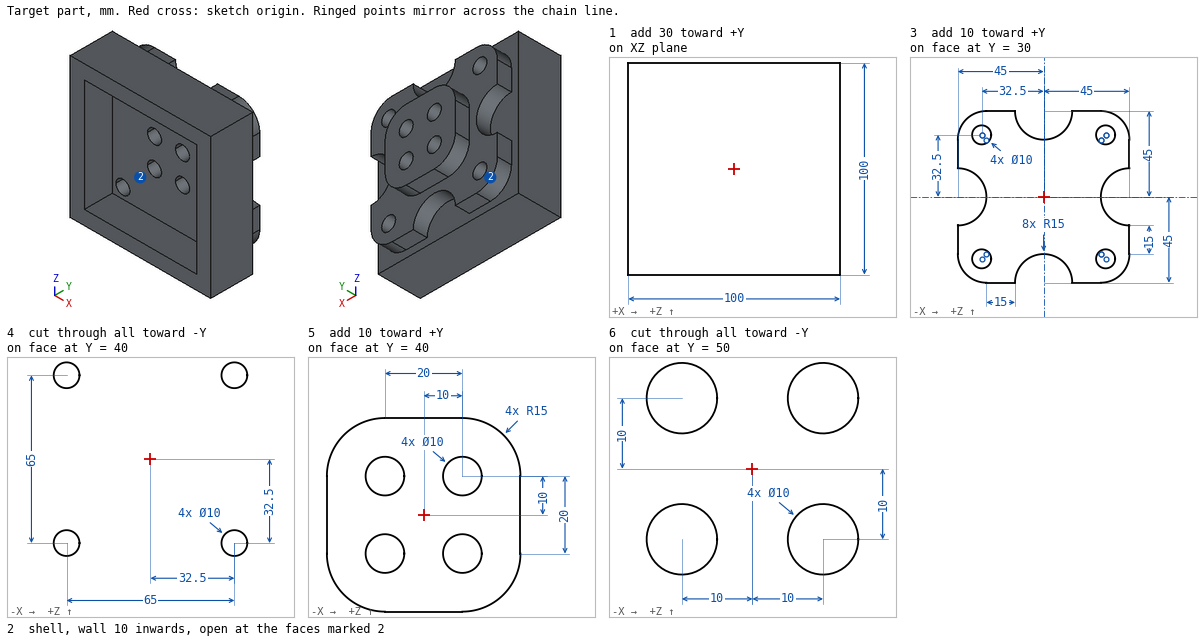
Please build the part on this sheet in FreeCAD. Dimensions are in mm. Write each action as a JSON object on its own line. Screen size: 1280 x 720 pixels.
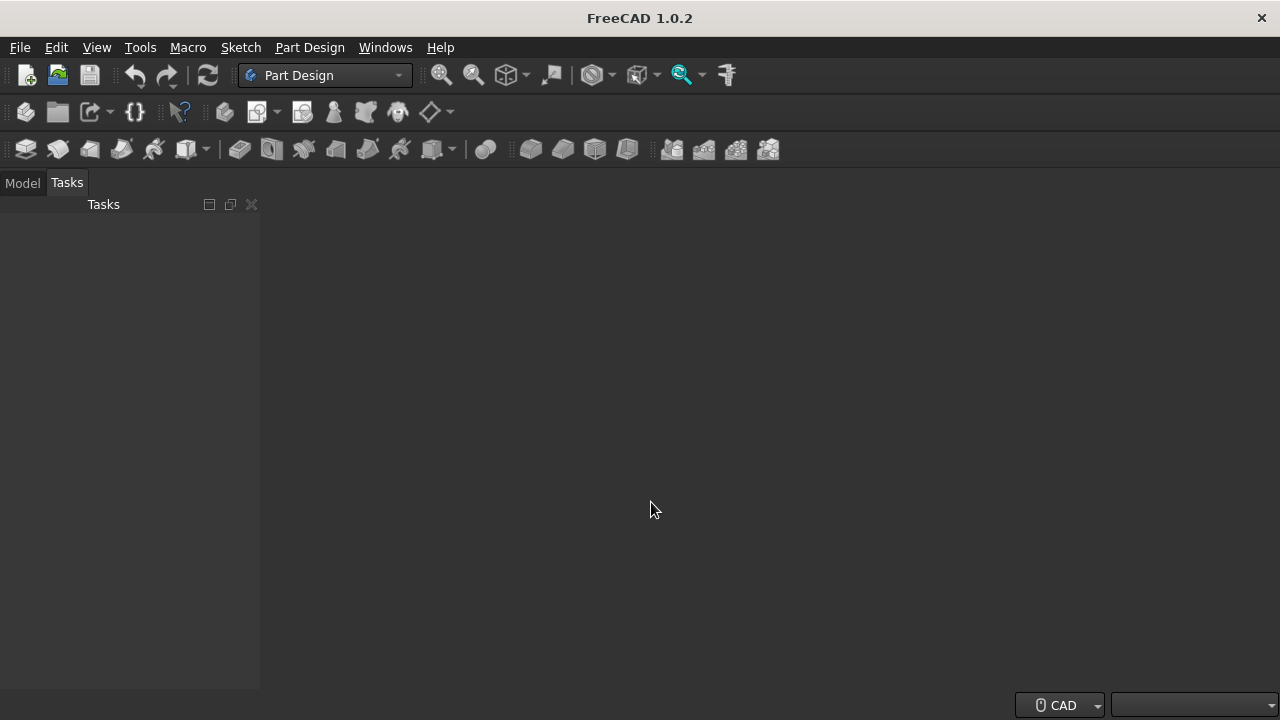
{"action": "left_click", "coordinate": [26, 76]}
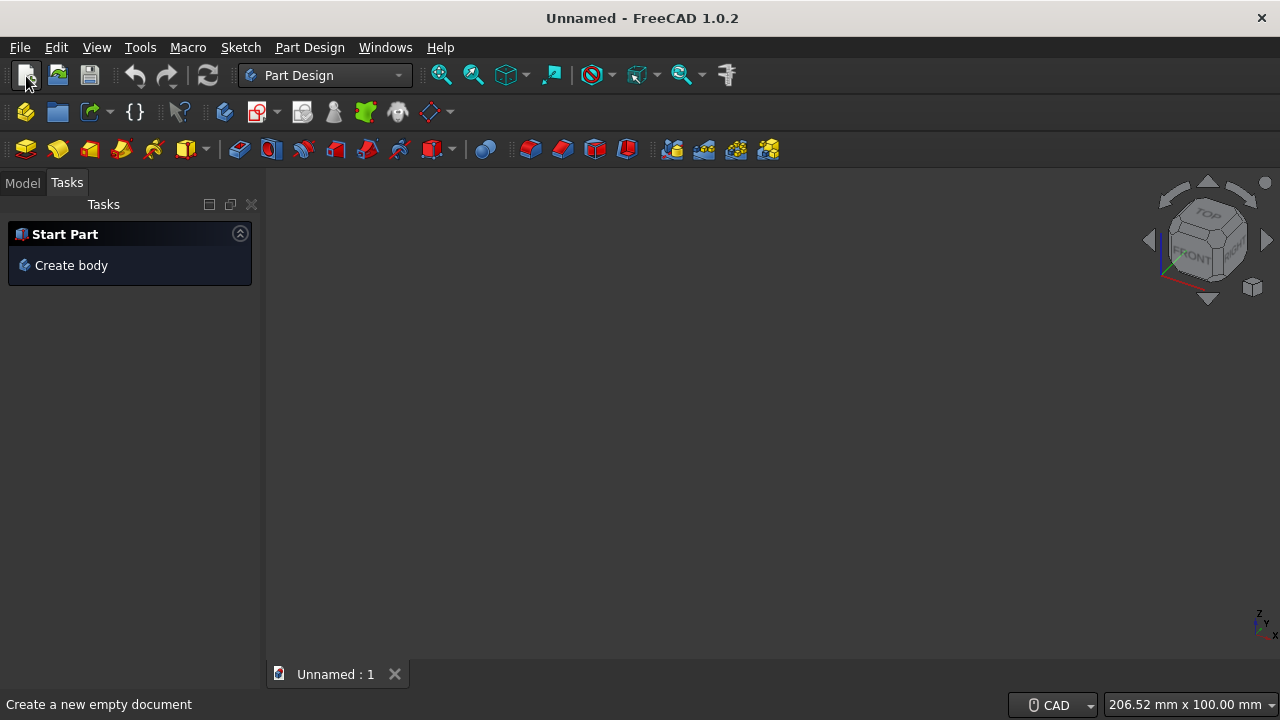
{"action": "left_click", "coordinate": [258, 112]}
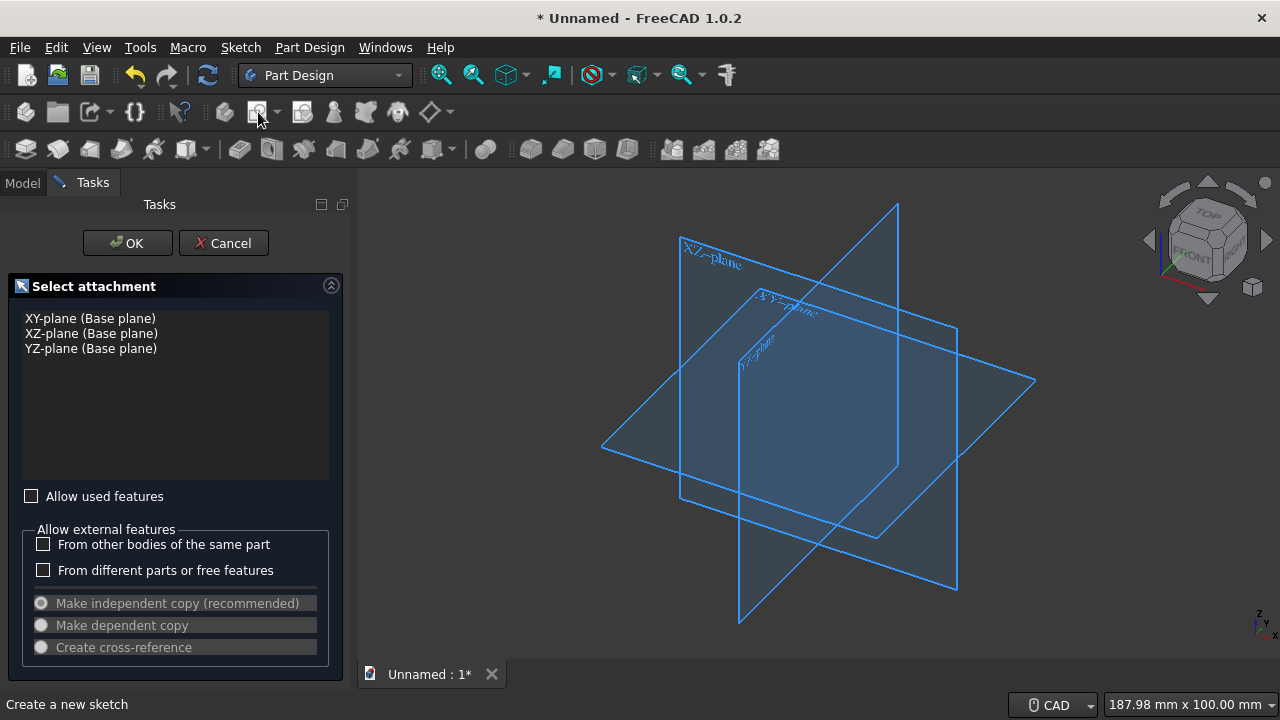
{"action": "left_click", "coordinate": [82, 334]}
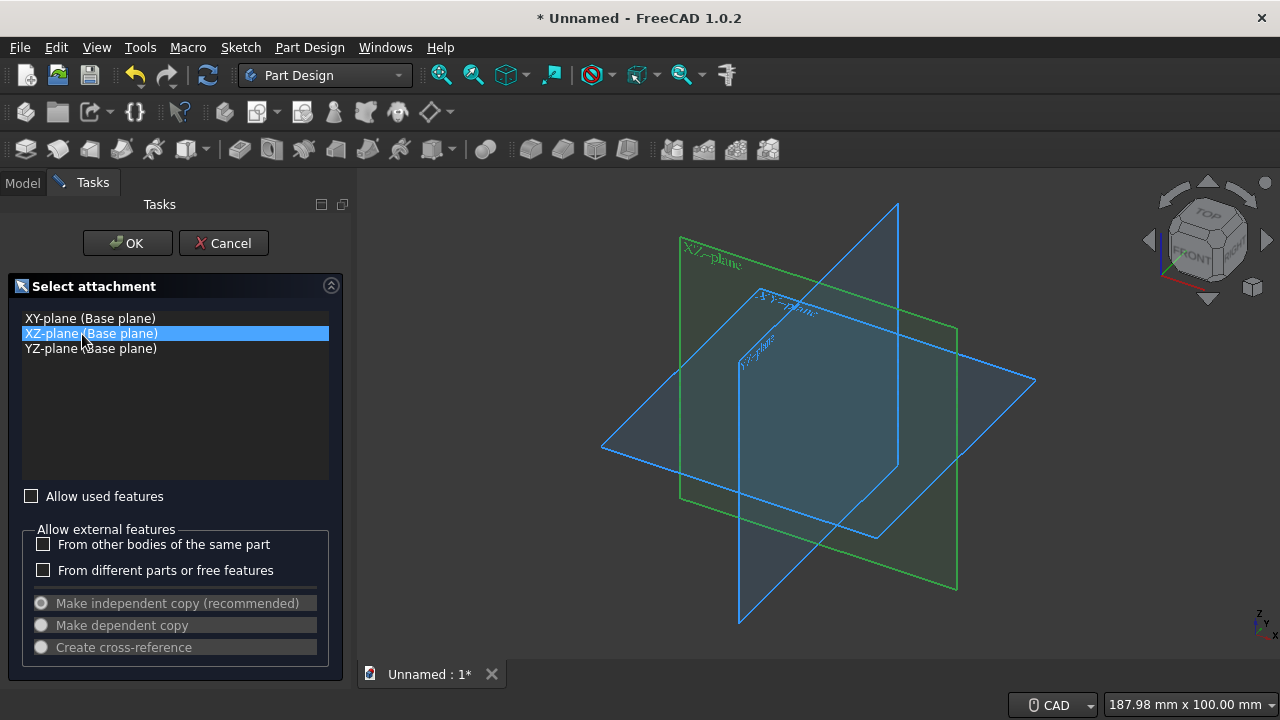
{"action": "left_click", "coordinate": [128, 243]}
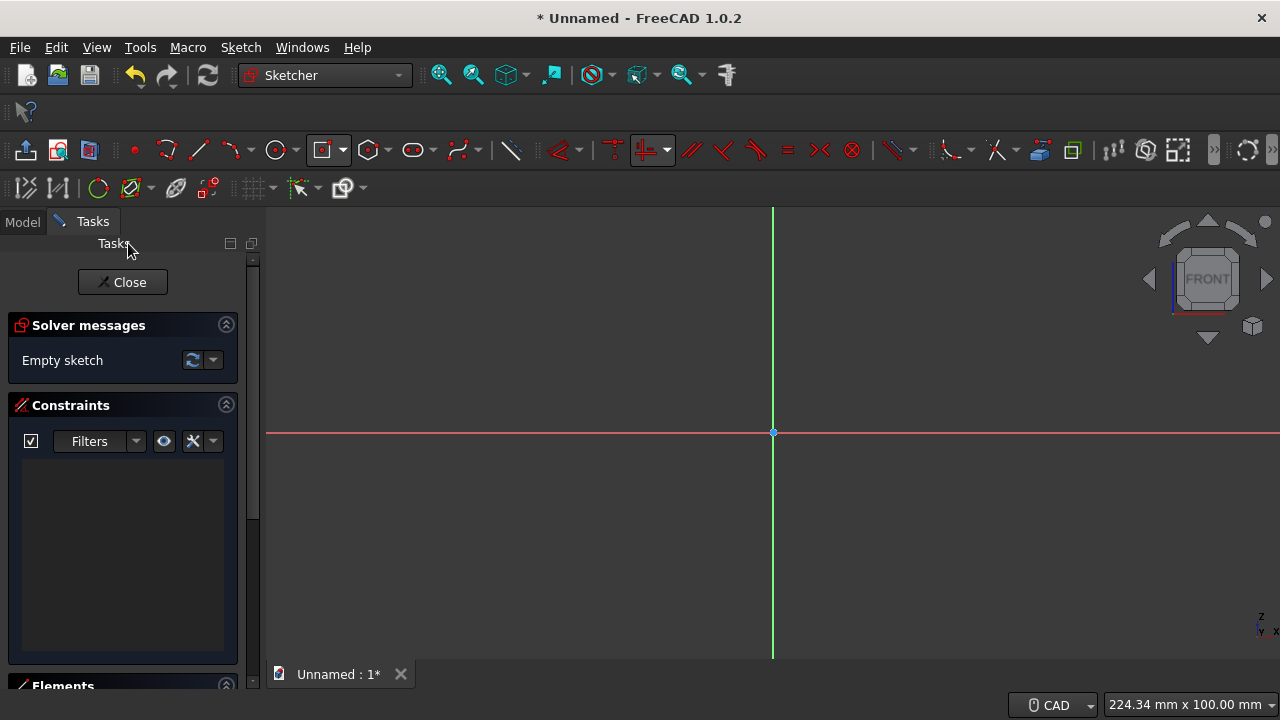
{"action": "scroll", "coordinate": [565, 433], "scroll_direction": "down", "scroll_amount": 2}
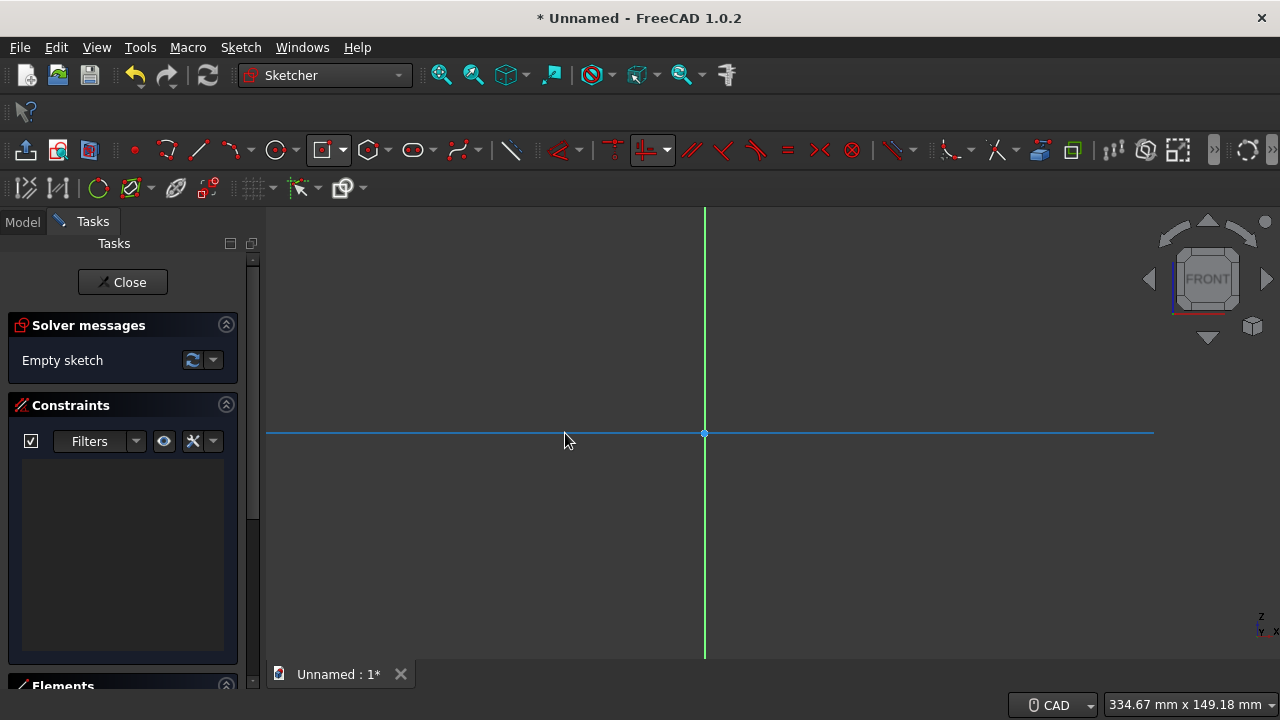
{"action": "left_click", "coordinate": [322, 150]}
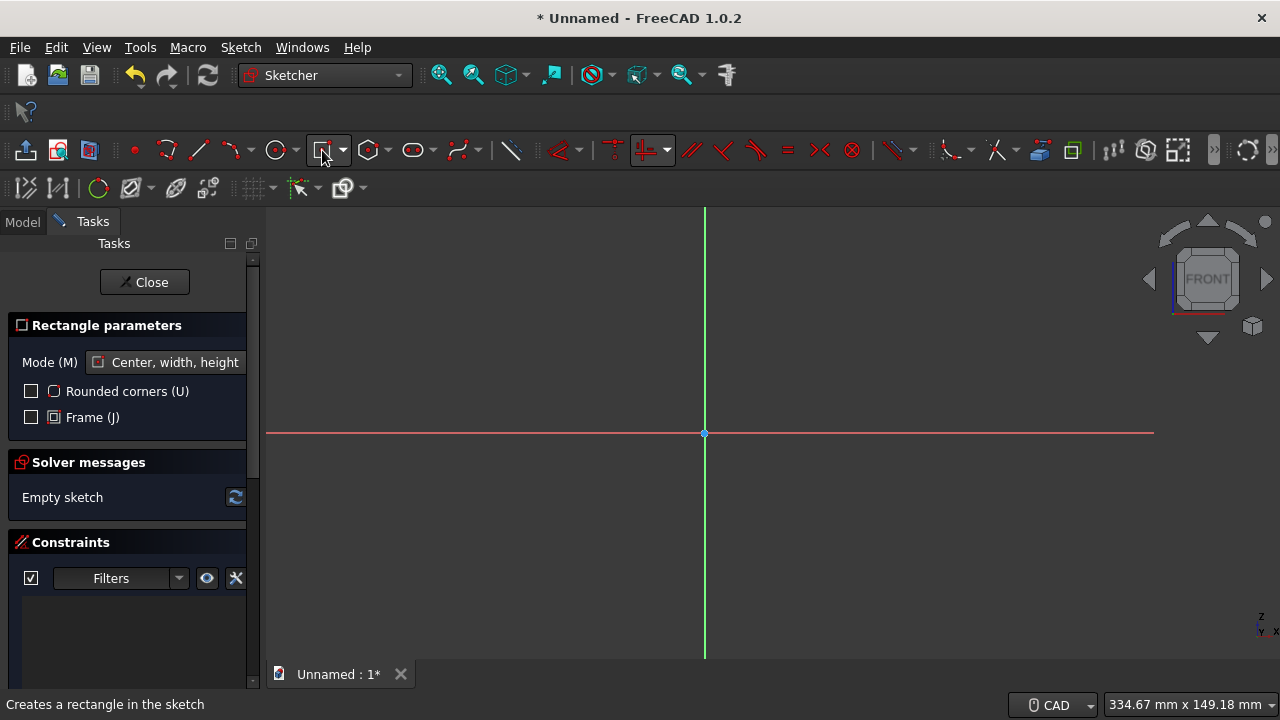
{"action": "left_click", "coordinate": [705, 433]}
{"action": "left_click", "coordinate": [856, 282]}
{"action": "key", "text": "Escape"}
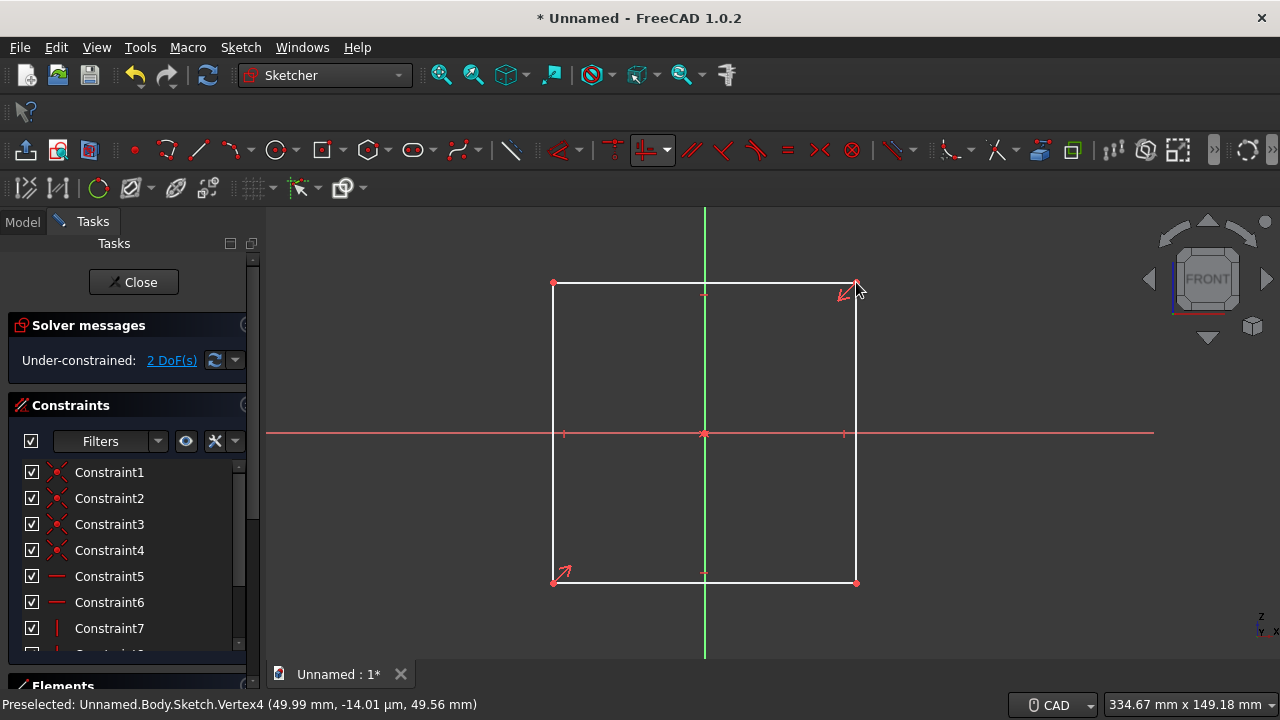
{"action": "left_click", "coordinate": [558, 150]}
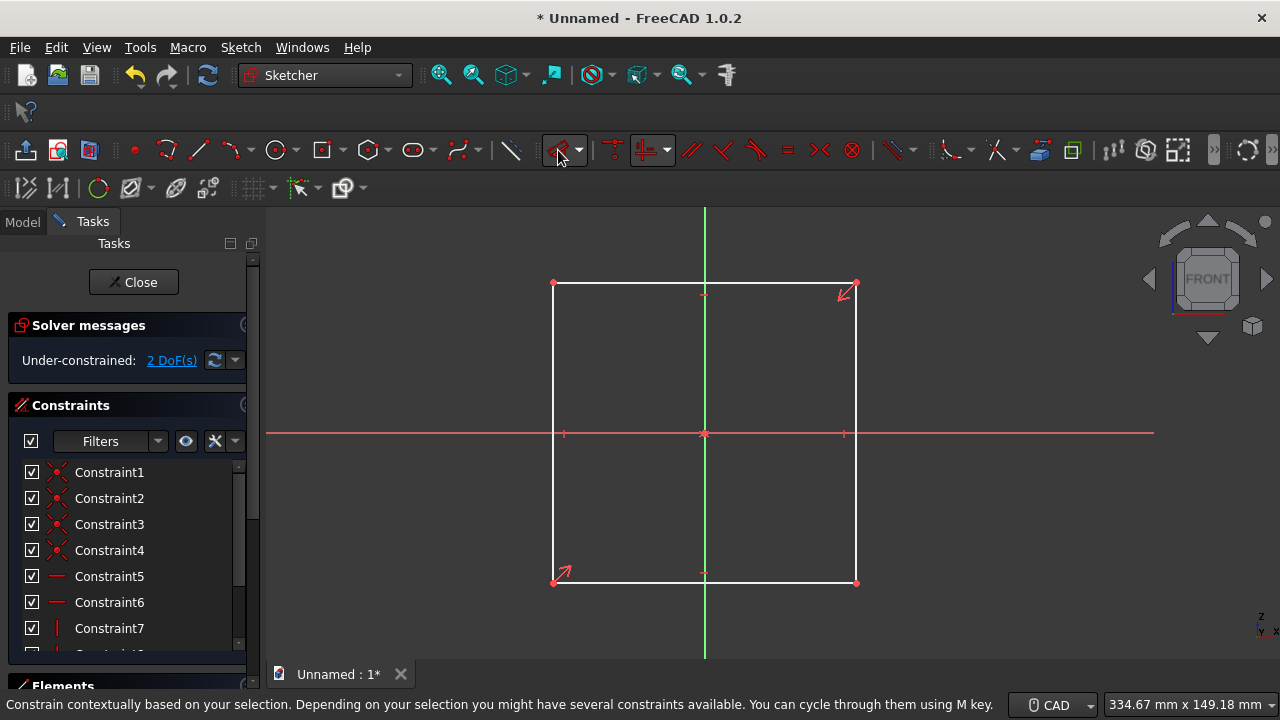
{"action": "left_click", "coordinate": [644, 583]}
{"action": "left_click", "coordinate": [635, 617]}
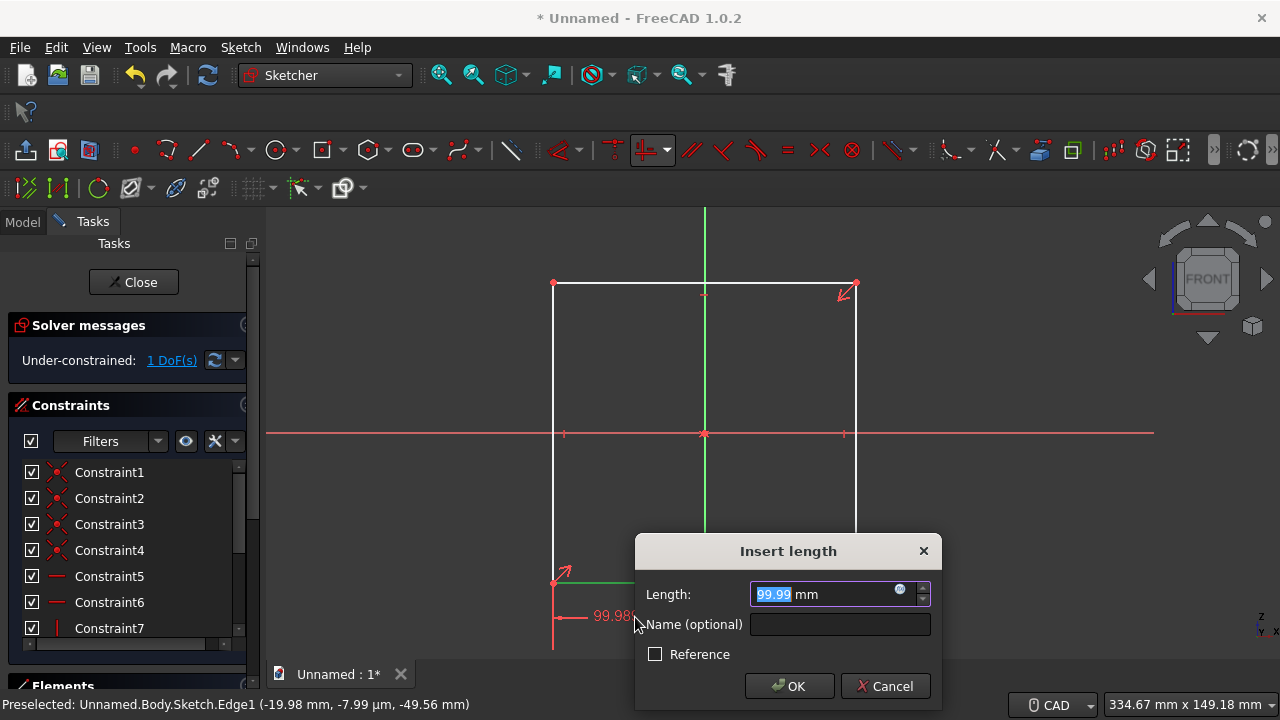
{"action": "type", "text": "100"}
{"action": "key", "text": "Return"}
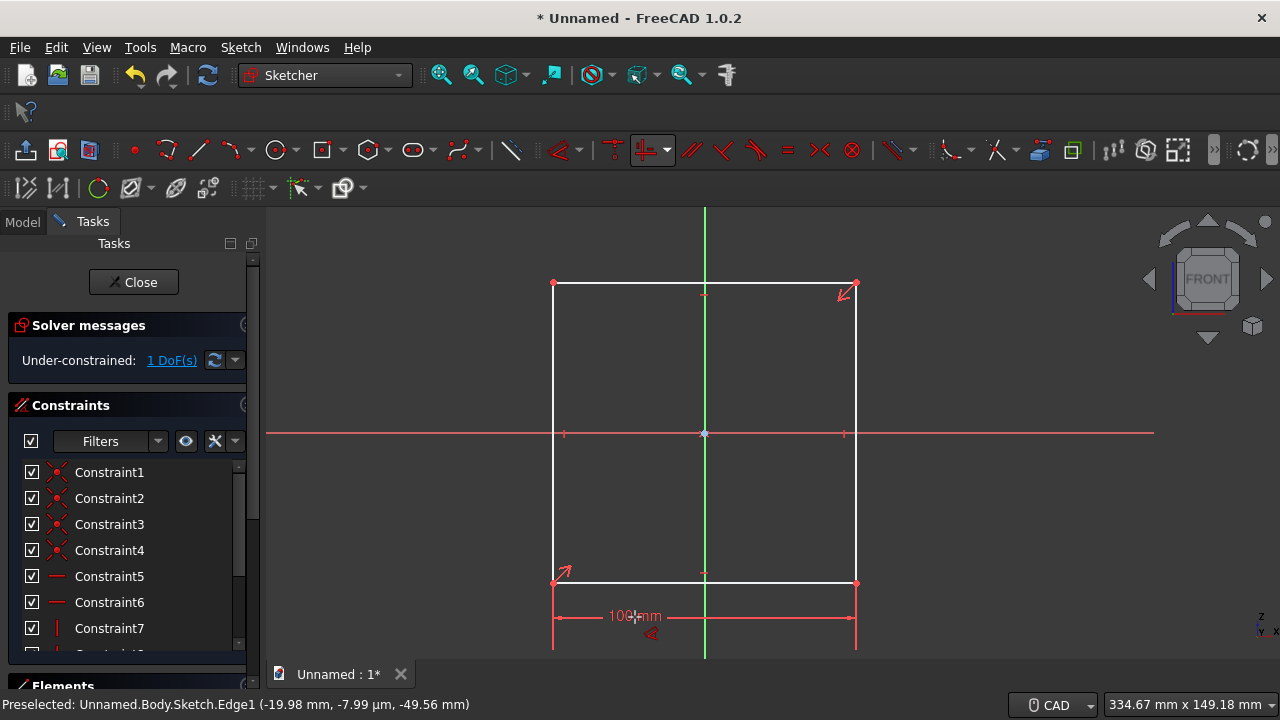
{"action": "left_click", "coordinate": [856, 493]}
{"action": "left_click", "coordinate": [890, 364]}